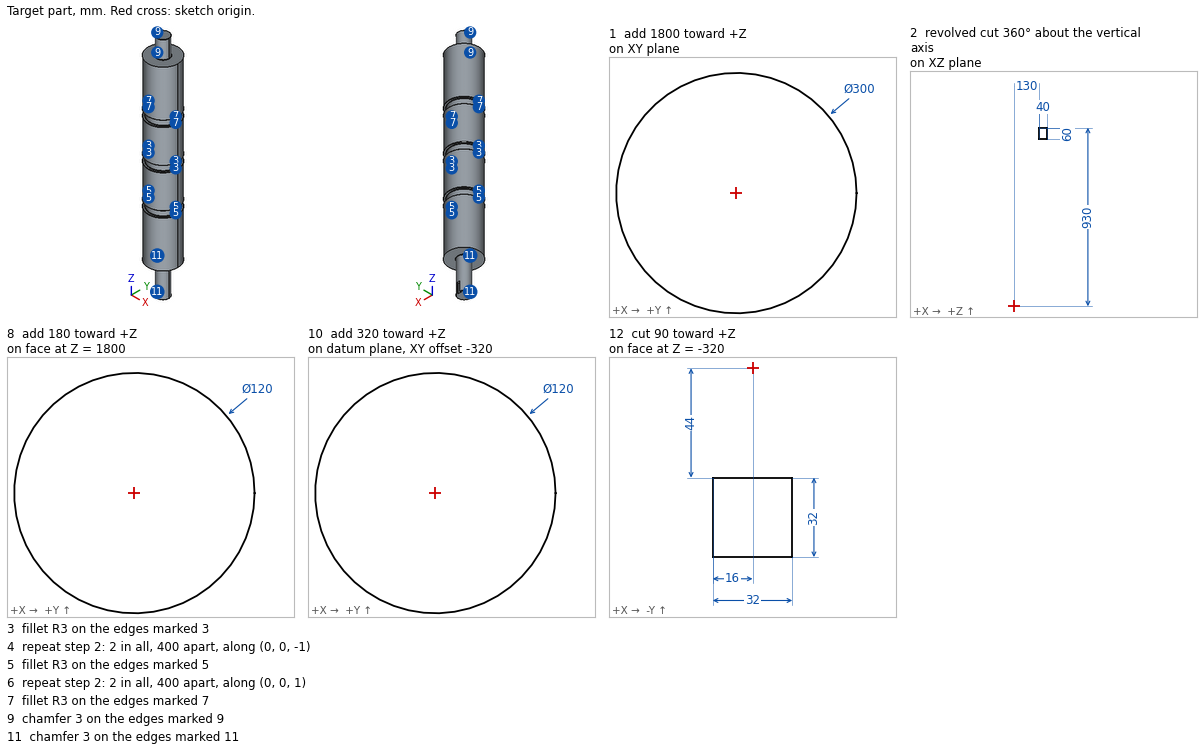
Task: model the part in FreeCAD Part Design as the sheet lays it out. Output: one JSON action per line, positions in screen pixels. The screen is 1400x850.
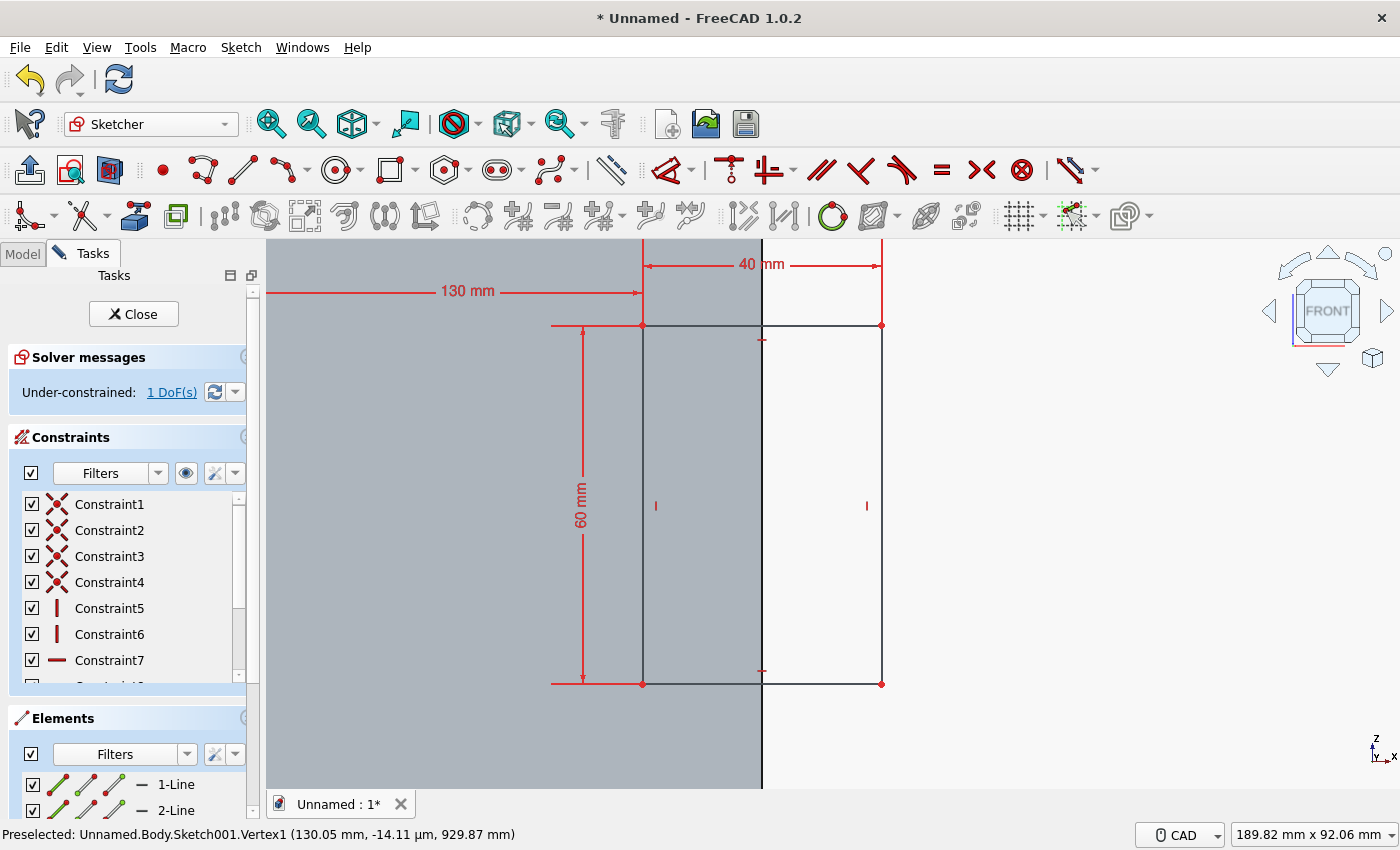
{"action": "left_click", "coordinate": [643, 326]}
{"action": "left_click", "coordinate": [677, 543]}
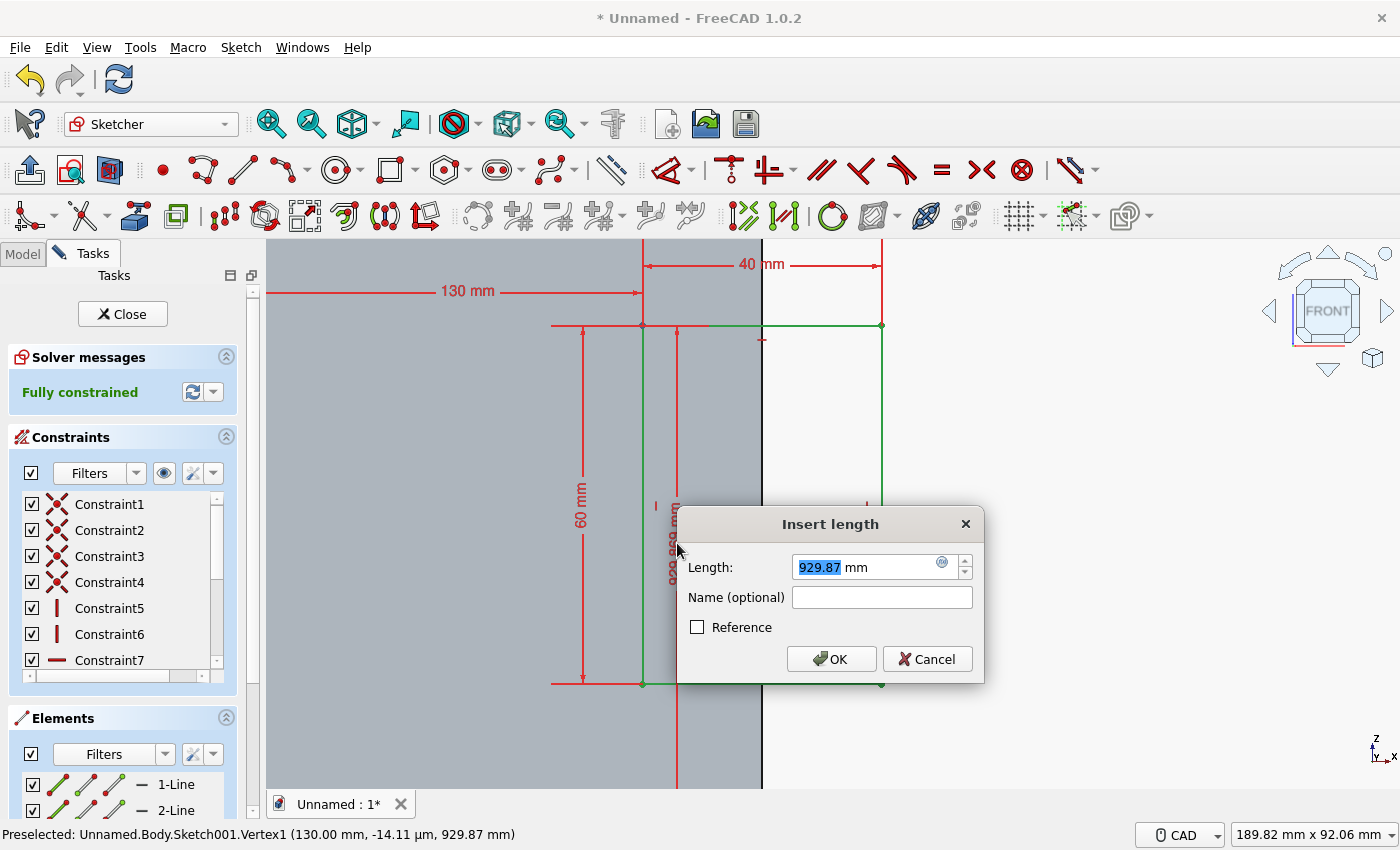
{"action": "type", "text": "930"}
{"action": "key", "text": "Return"}
{"action": "key", "text": "Escape"}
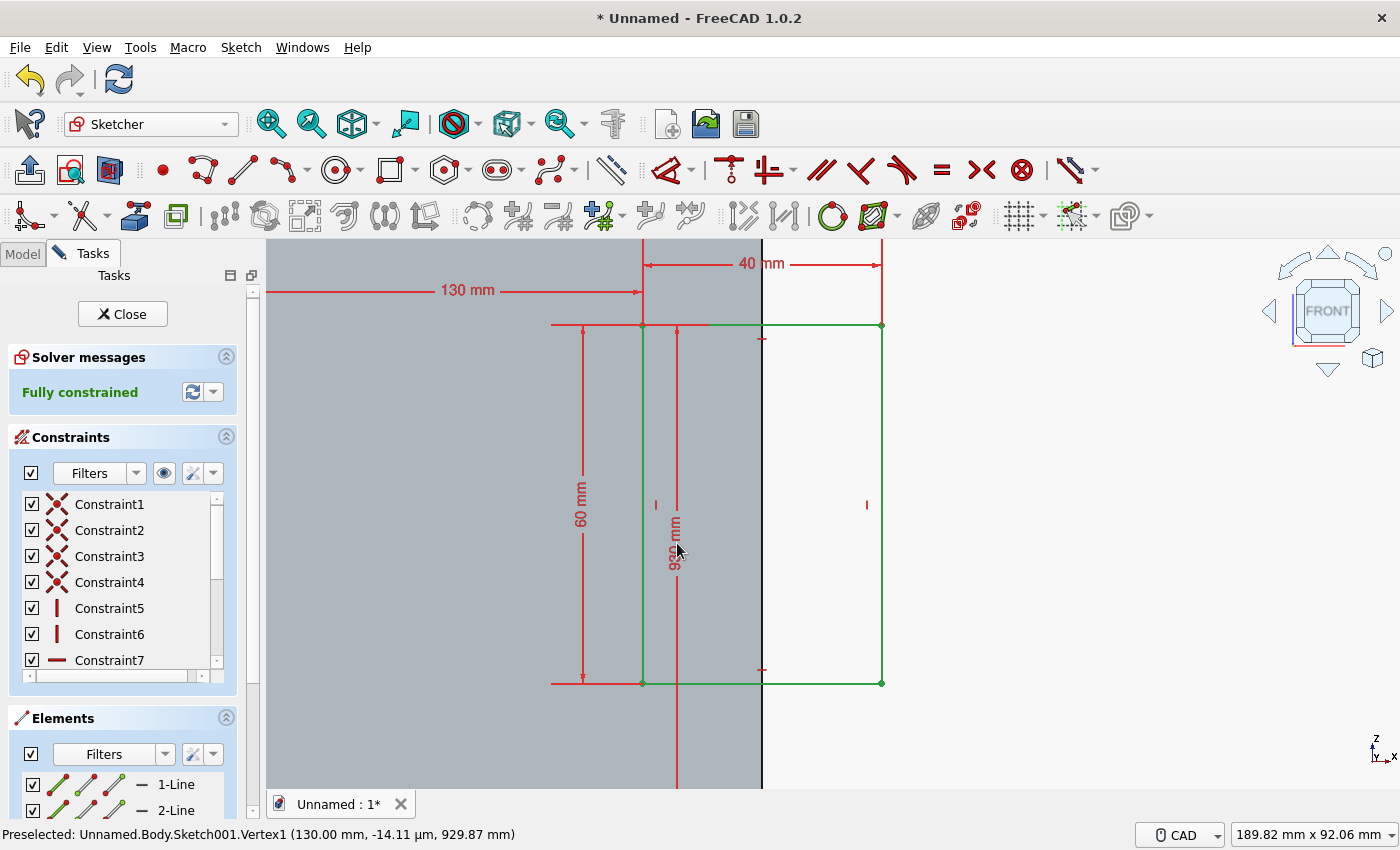
{"action": "left_click", "coordinate": [123, 314]}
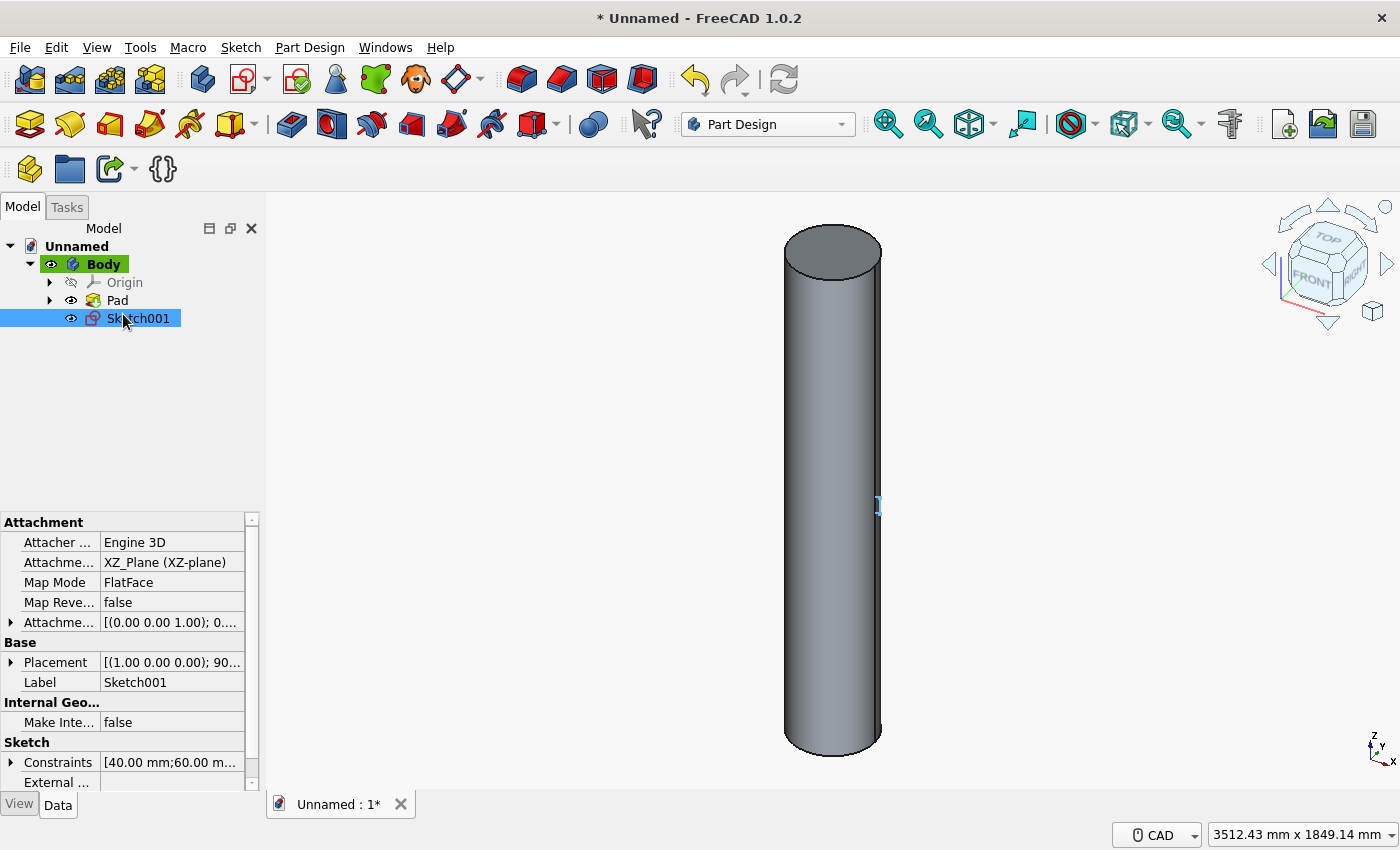
{"action": "left_click", "coordinate": [372, 124]}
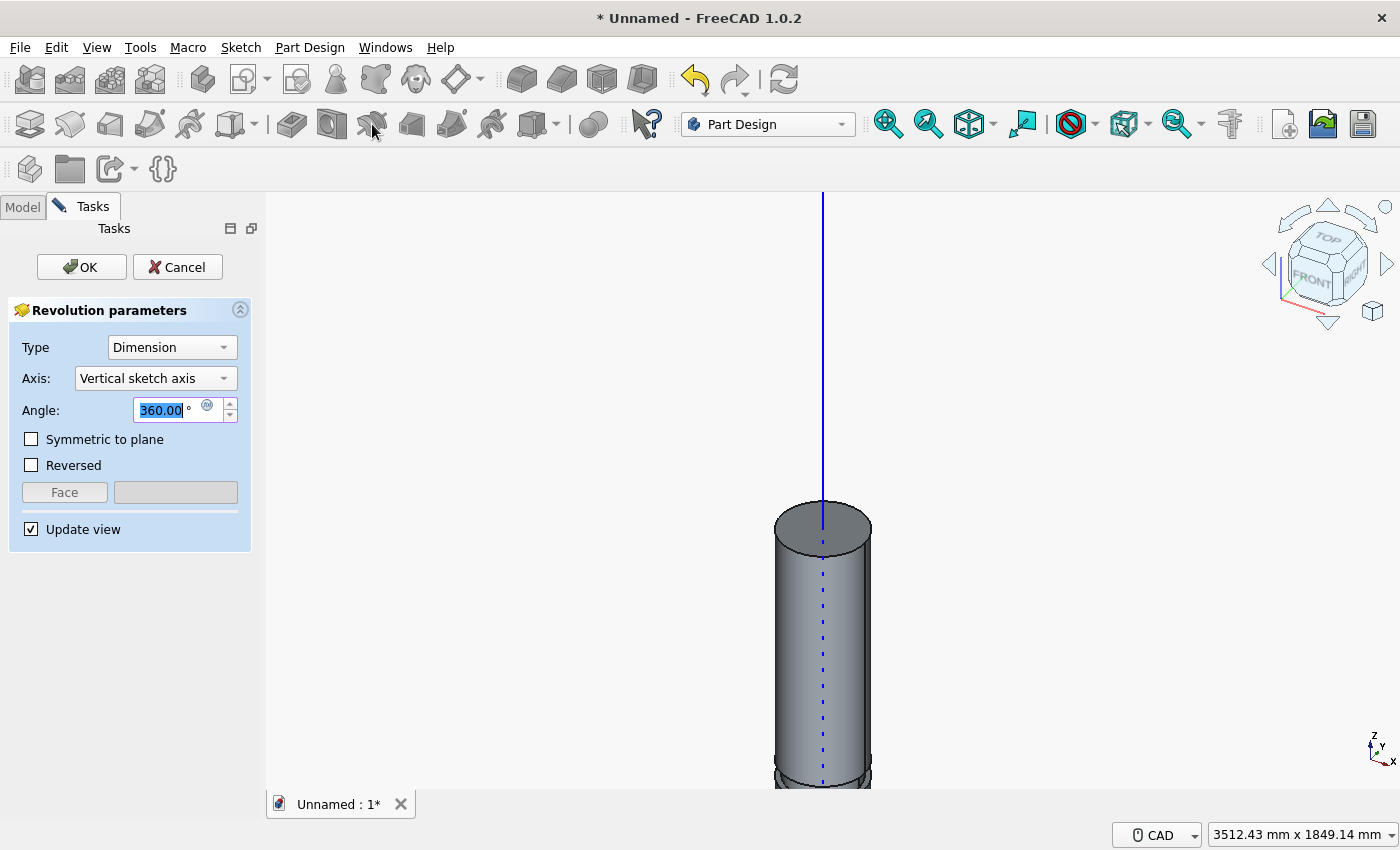
{"action": "left_click", "coordinate": [82, 267]}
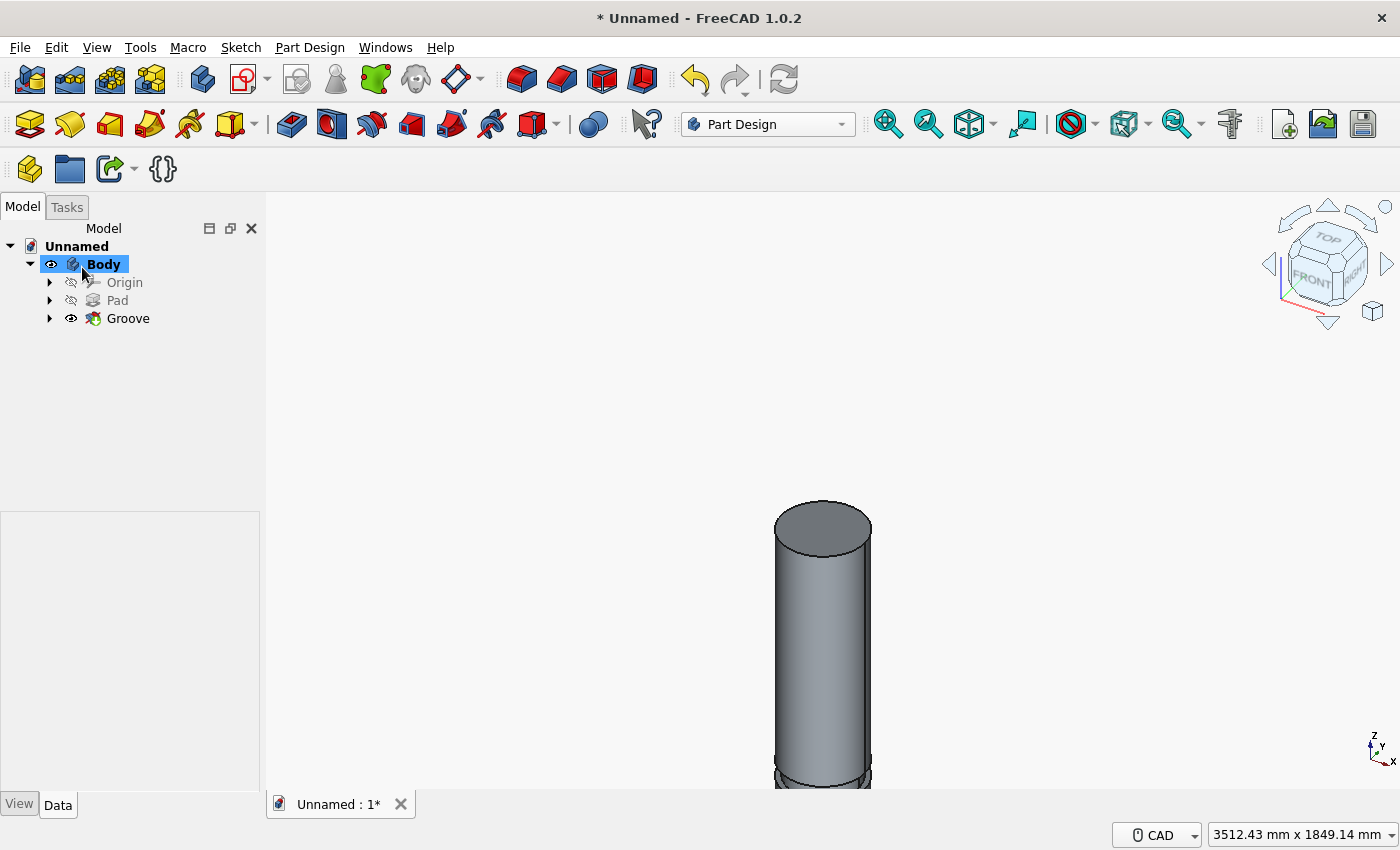
{"action": "left_click", "coordinate": [890, 124]}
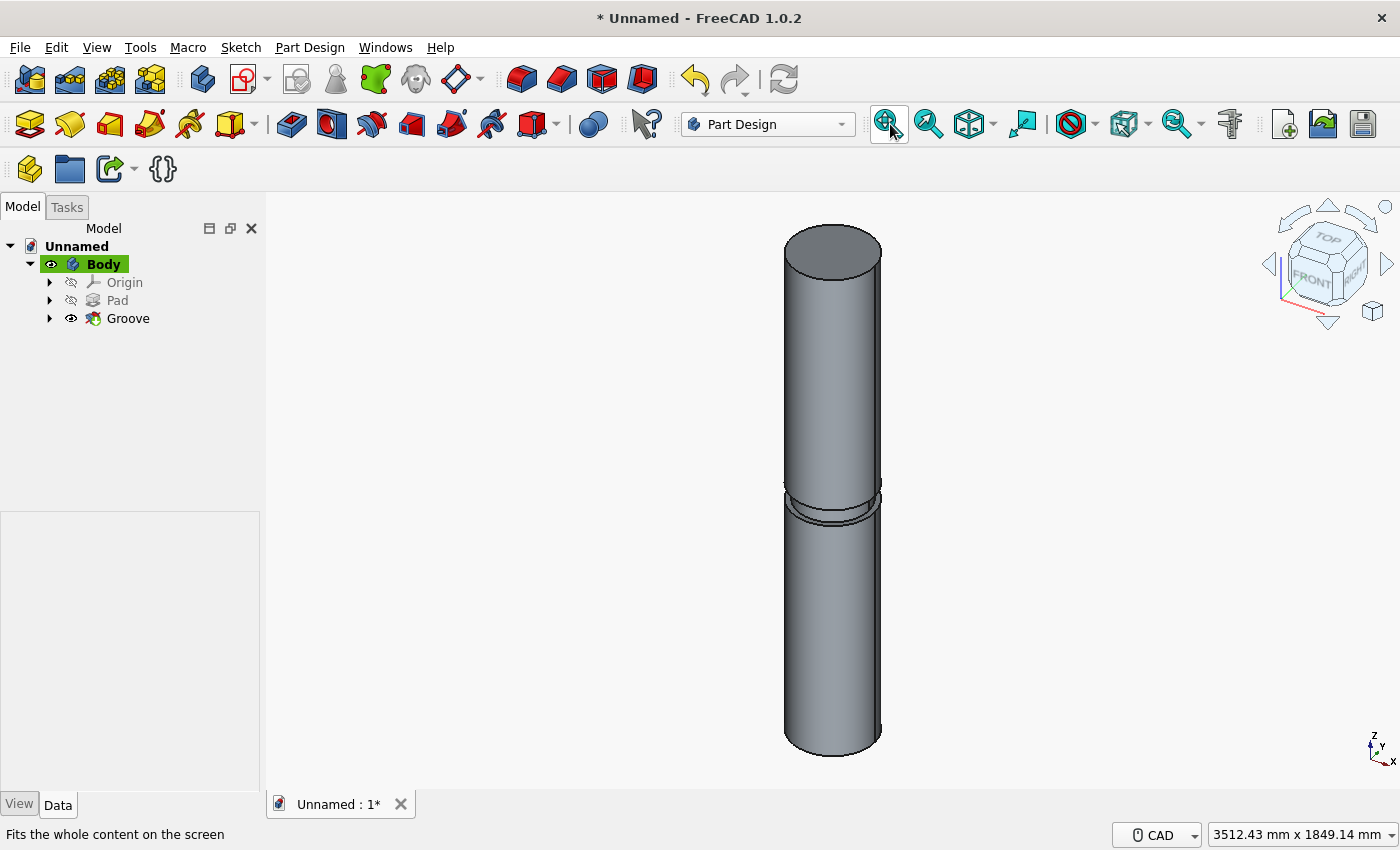
{"action": "left_click", "coordinate": [785, 500]}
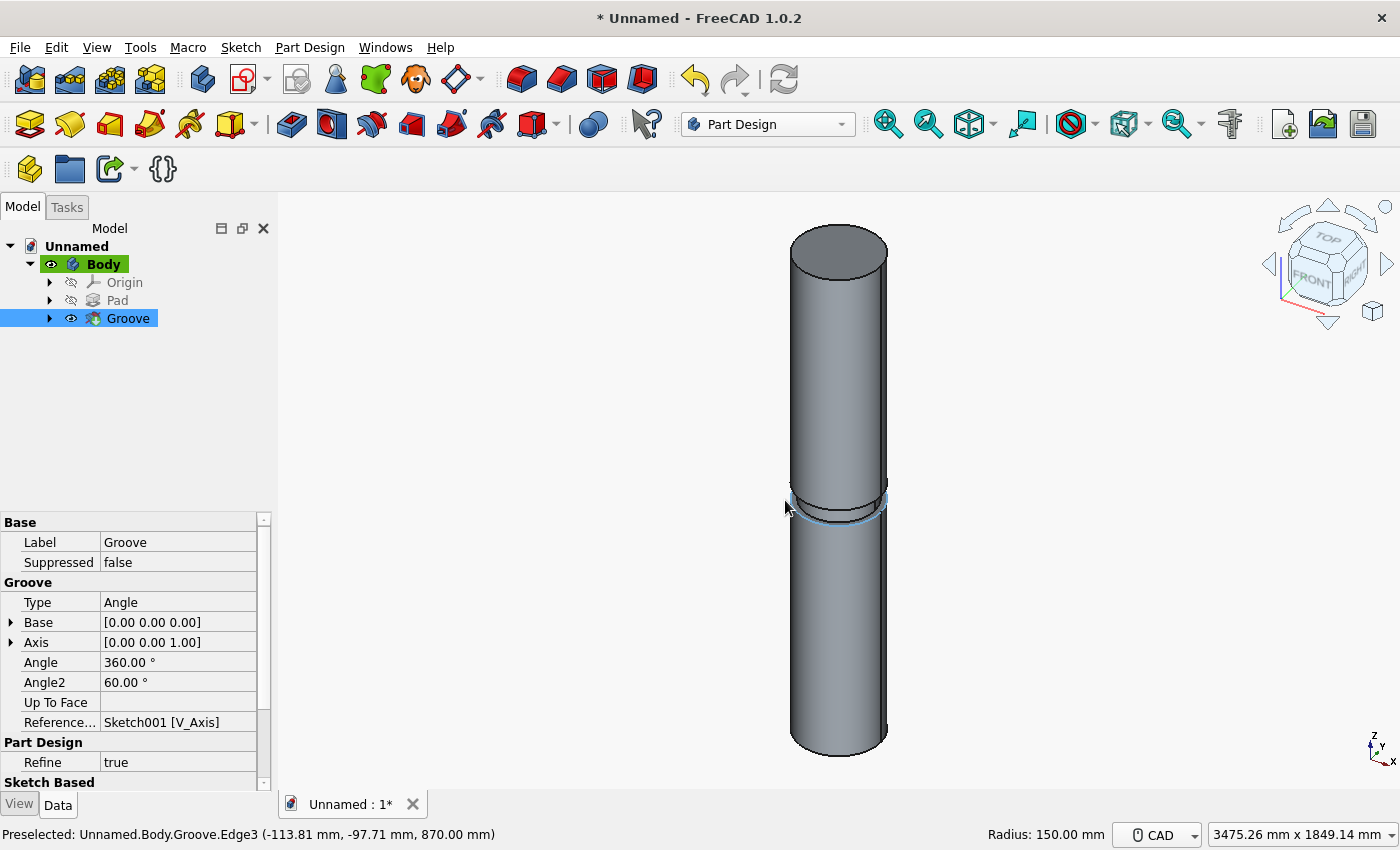
{"action": "key", "text": "0"}